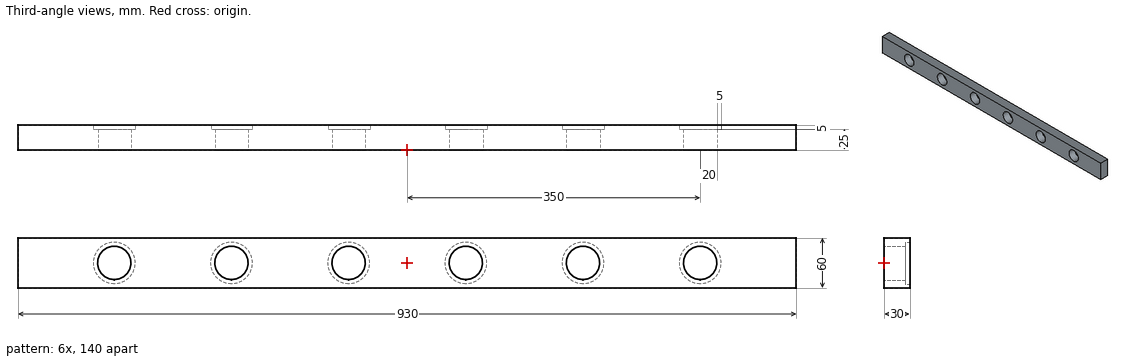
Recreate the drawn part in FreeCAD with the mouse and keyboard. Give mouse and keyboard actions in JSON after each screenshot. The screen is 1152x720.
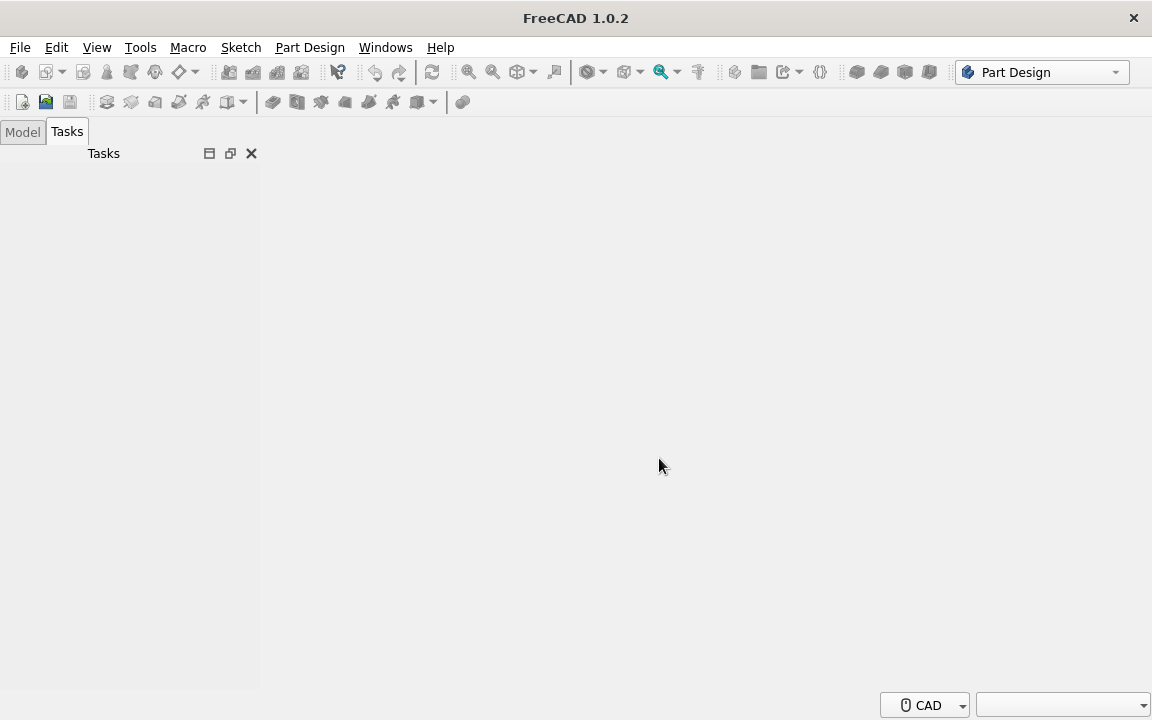
{"action": "left_click", "coordinate": [22, 102]}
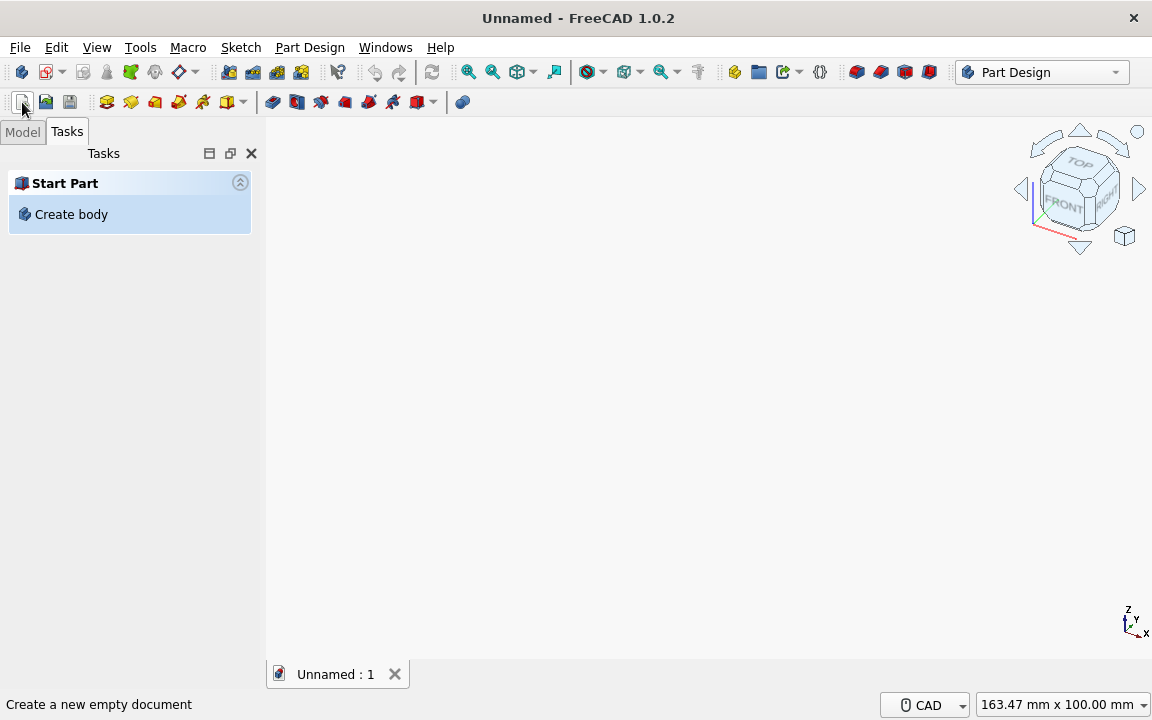
{"action": "left_click", "coordinate": [46, 72]}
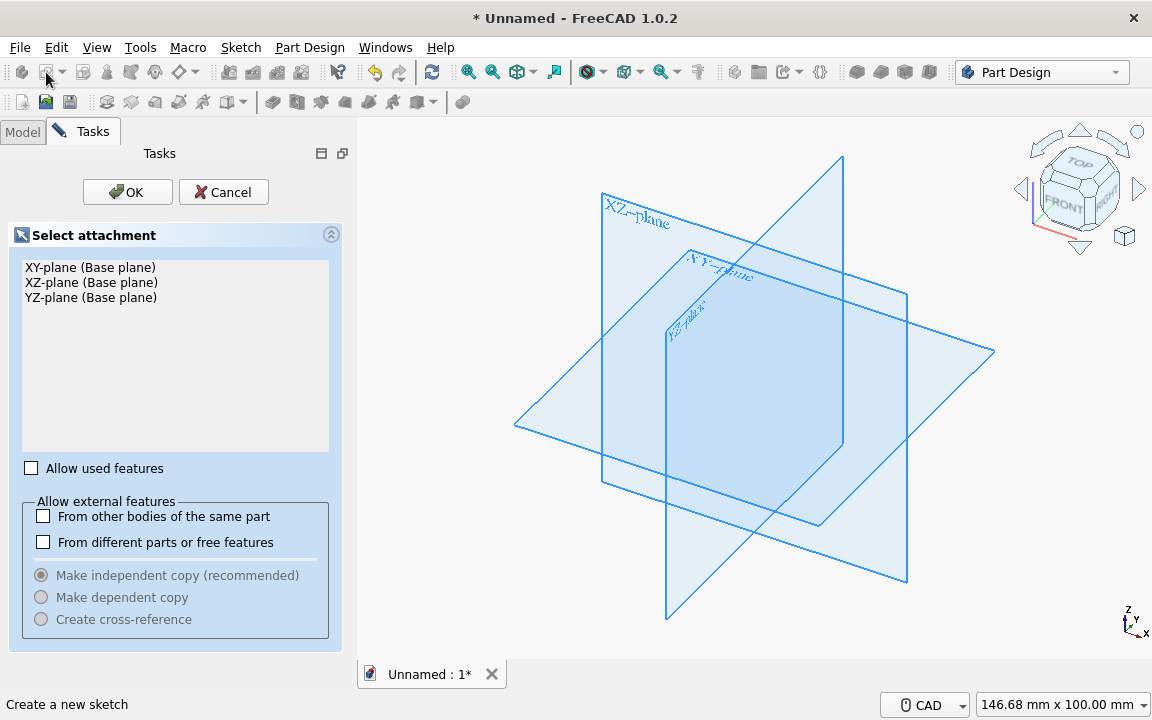
{"action": "left_click", "coordinate": [82, 282]}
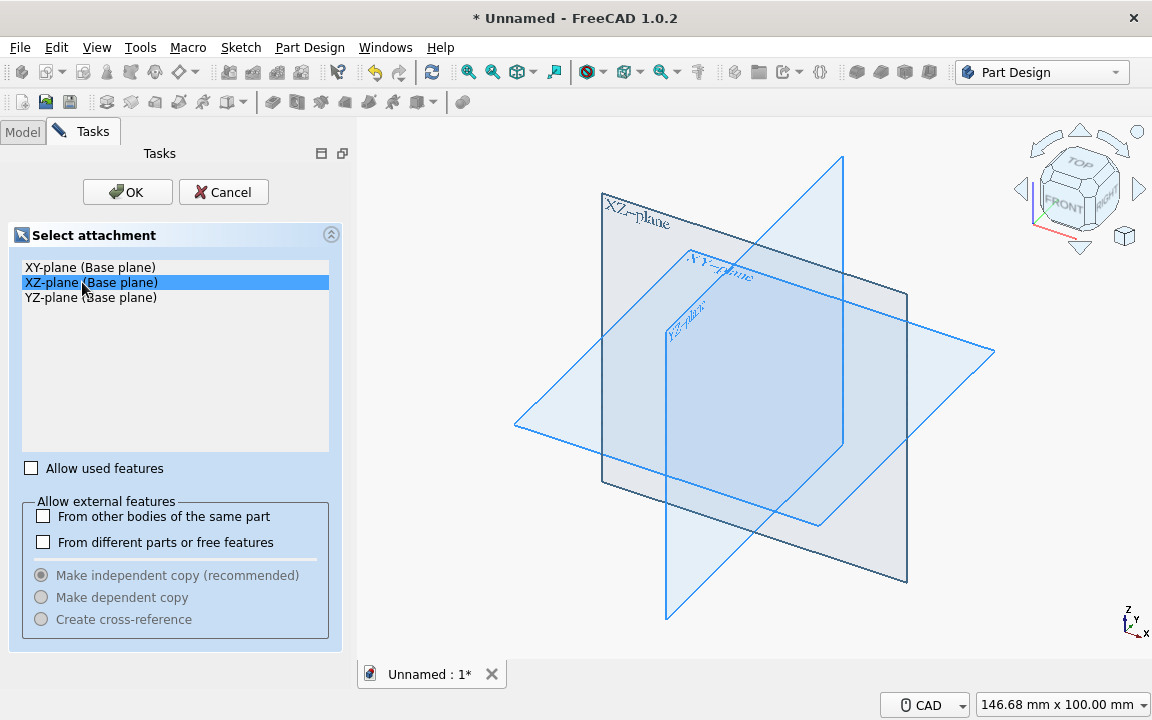
{"action": "left_click", "coordinate": [128, 192]}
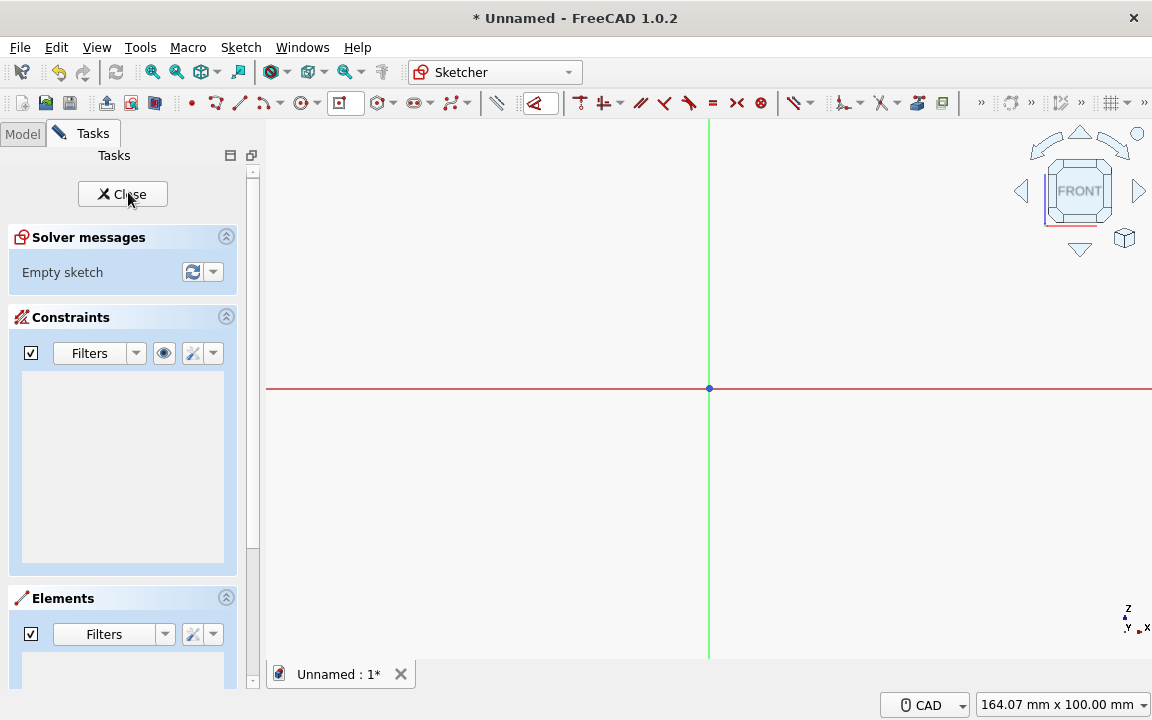
{"action": "scroll", "coordinate": [634, 389], "scroll_direction": "down", "scroll_amount": 12}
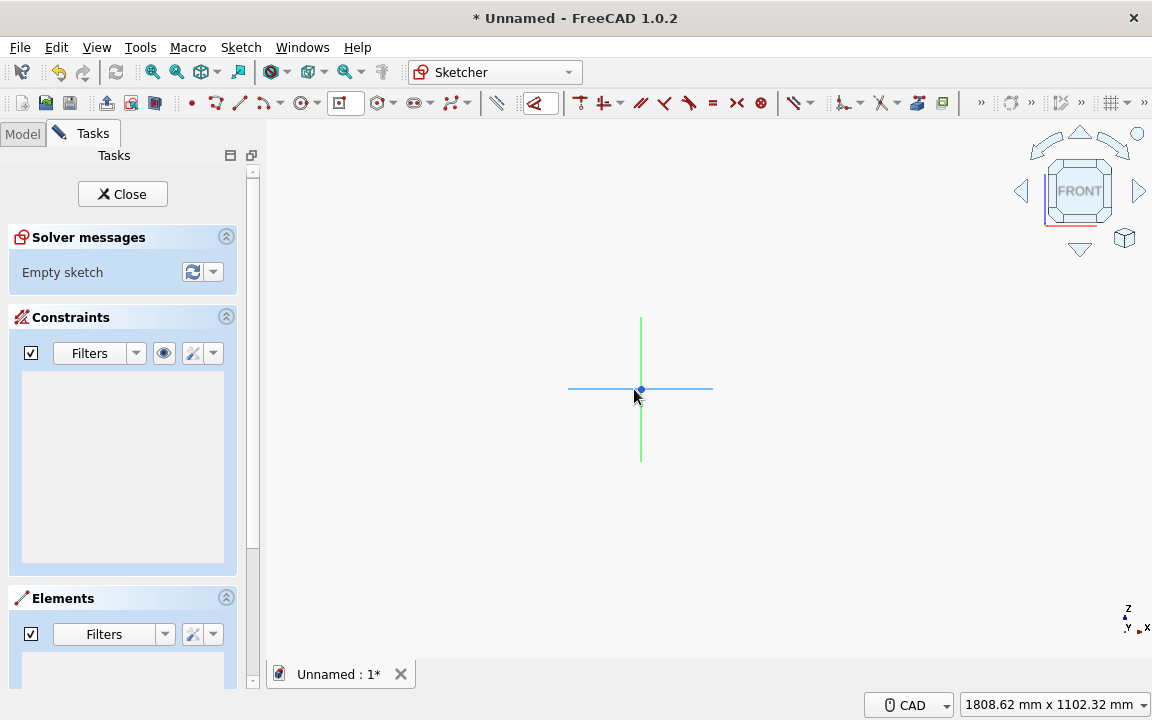
{"action": "left_click", "coordinate": [340, 104]}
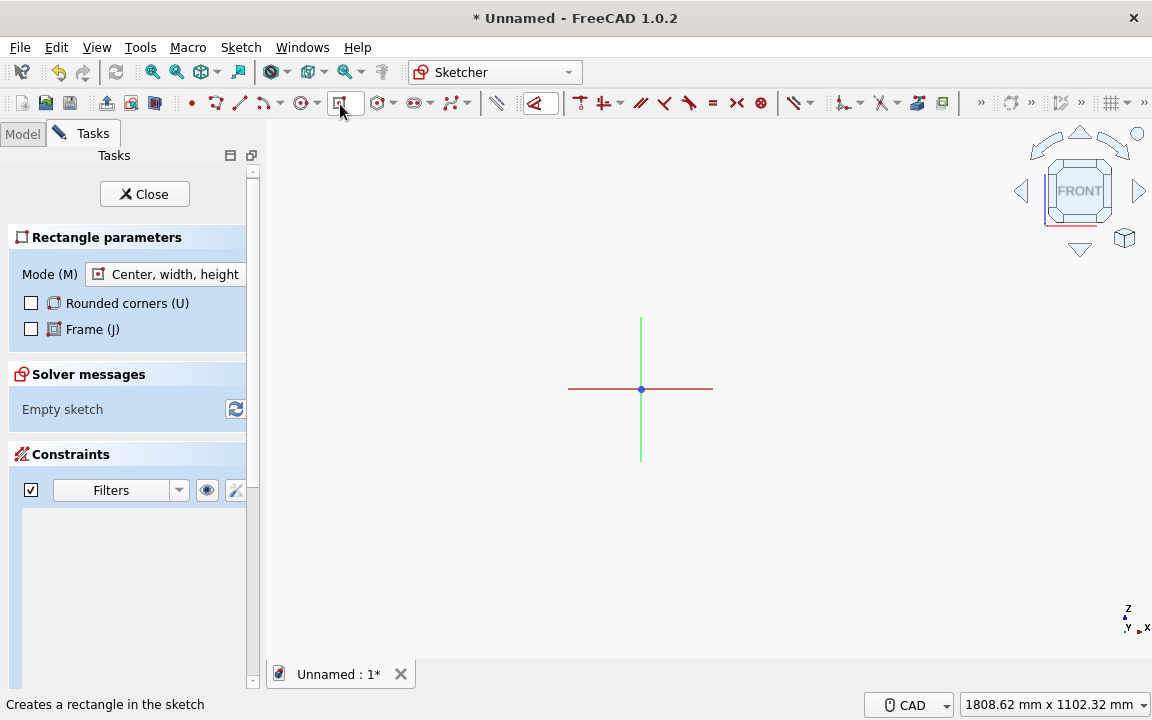
{"action": "left_click", "coordinate": [641, 389]}
{"action": "left_click", "coordinate": [869, 375]}
{"action": "key", "text": "Escape"}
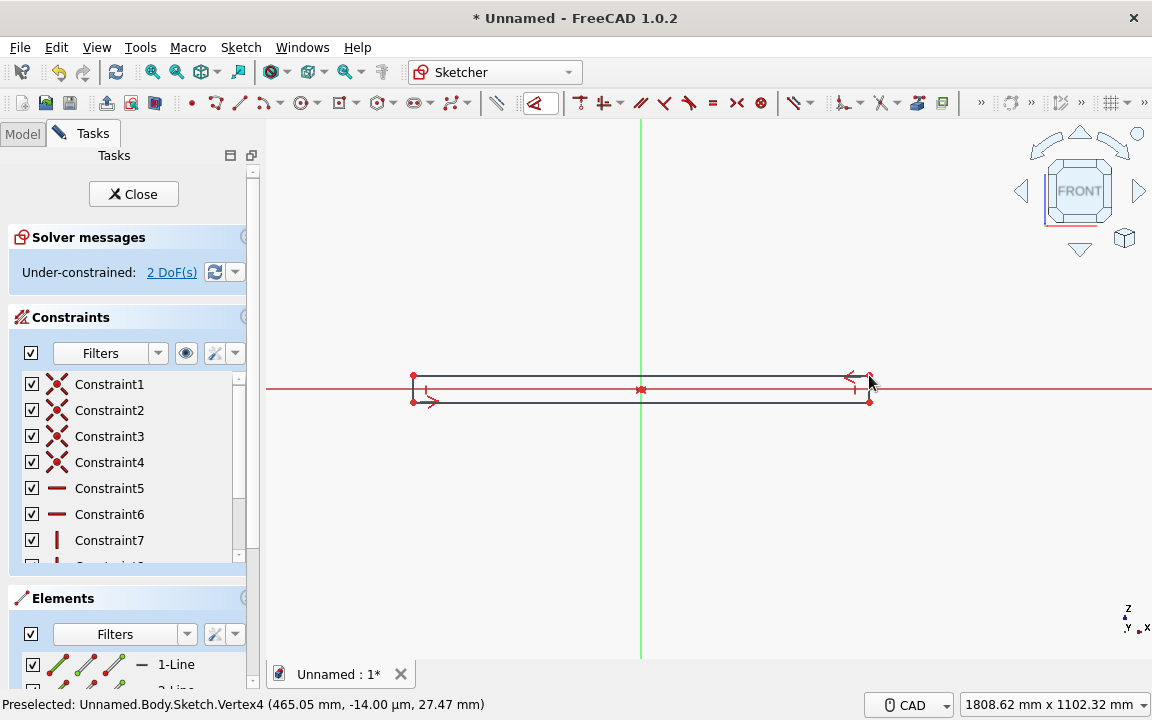
{"action": "left_click", "coordinate": [534, 104]}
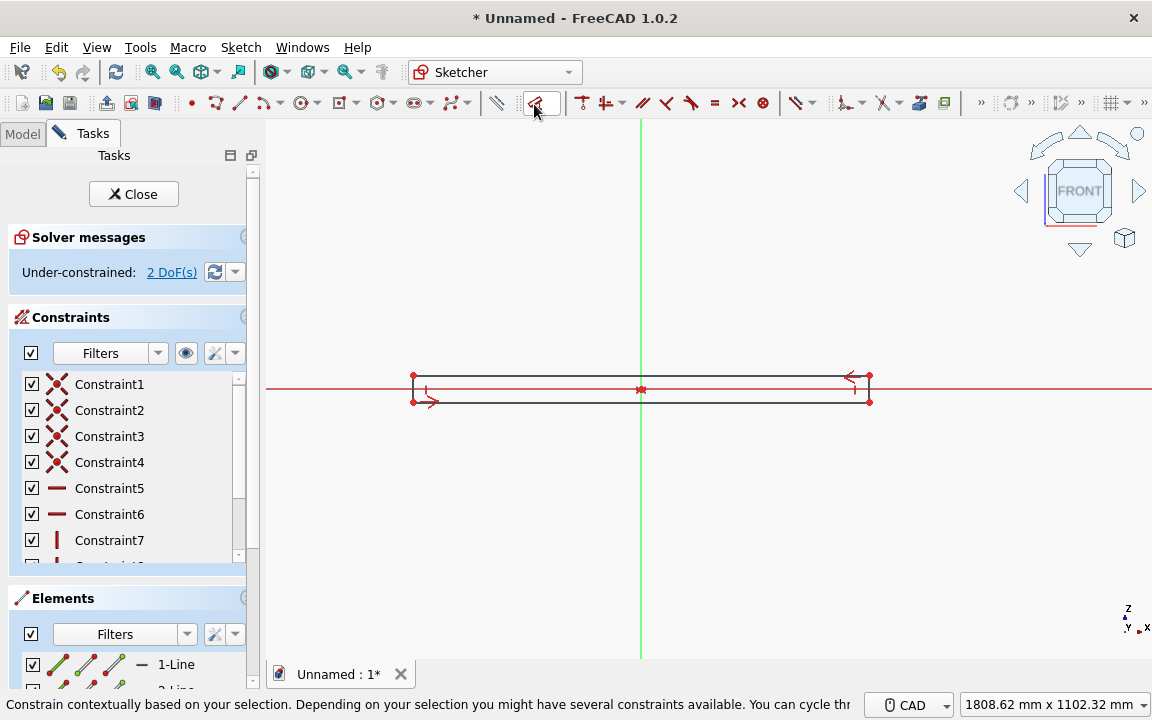
{"action": "scroll", "coordinate": [869, 392], "scroll_direction": "up", "scroll_amount": 2}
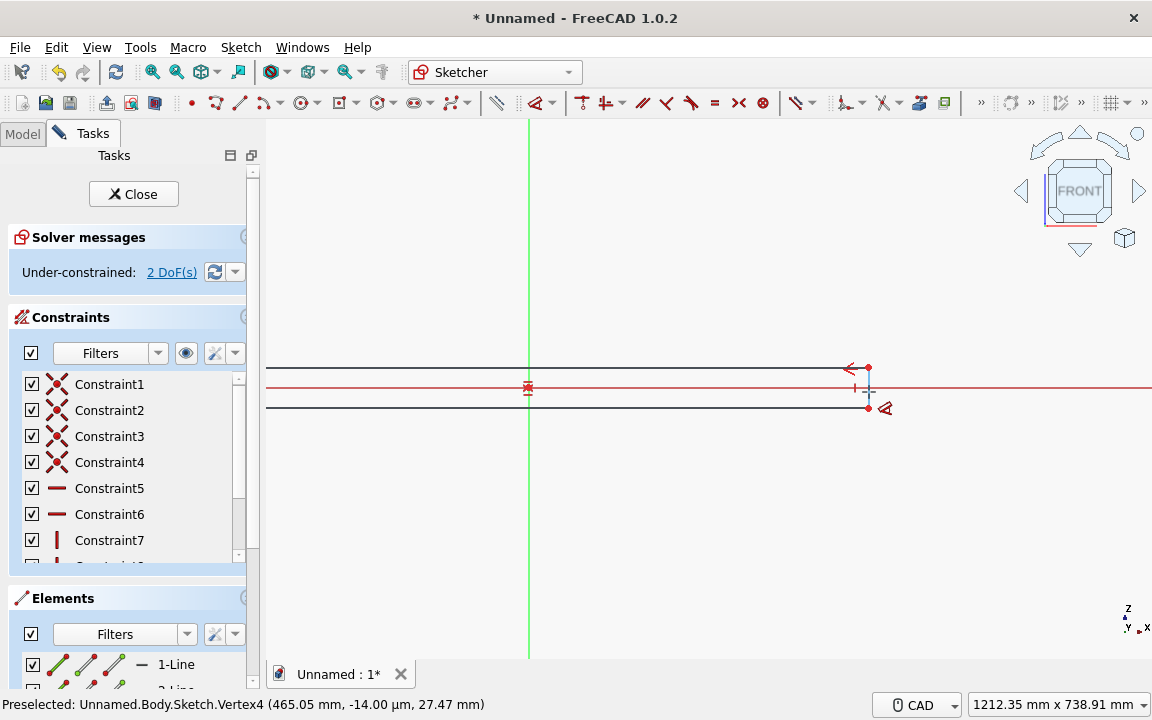
{"action": "left_click", "coordinate": [869, 392]}
{"action": "left_click", "coordinate": [903, 374]}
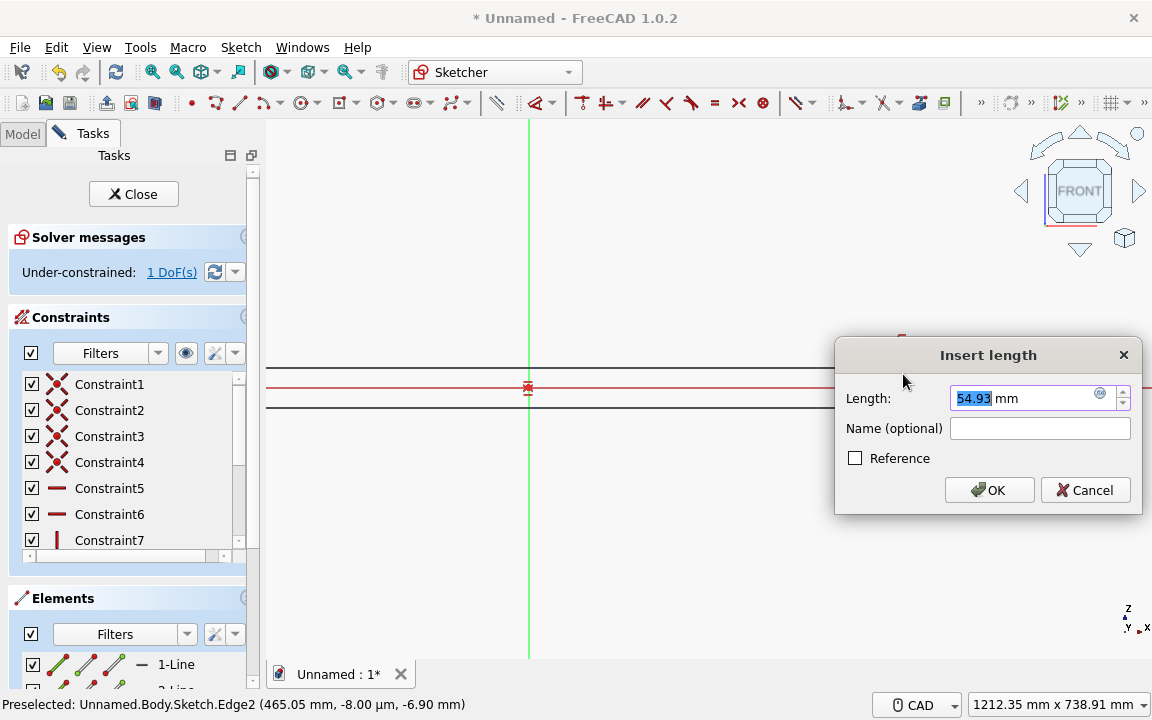
{"action": "type", "text": "60"}
{"action": "key", "text": "Return"}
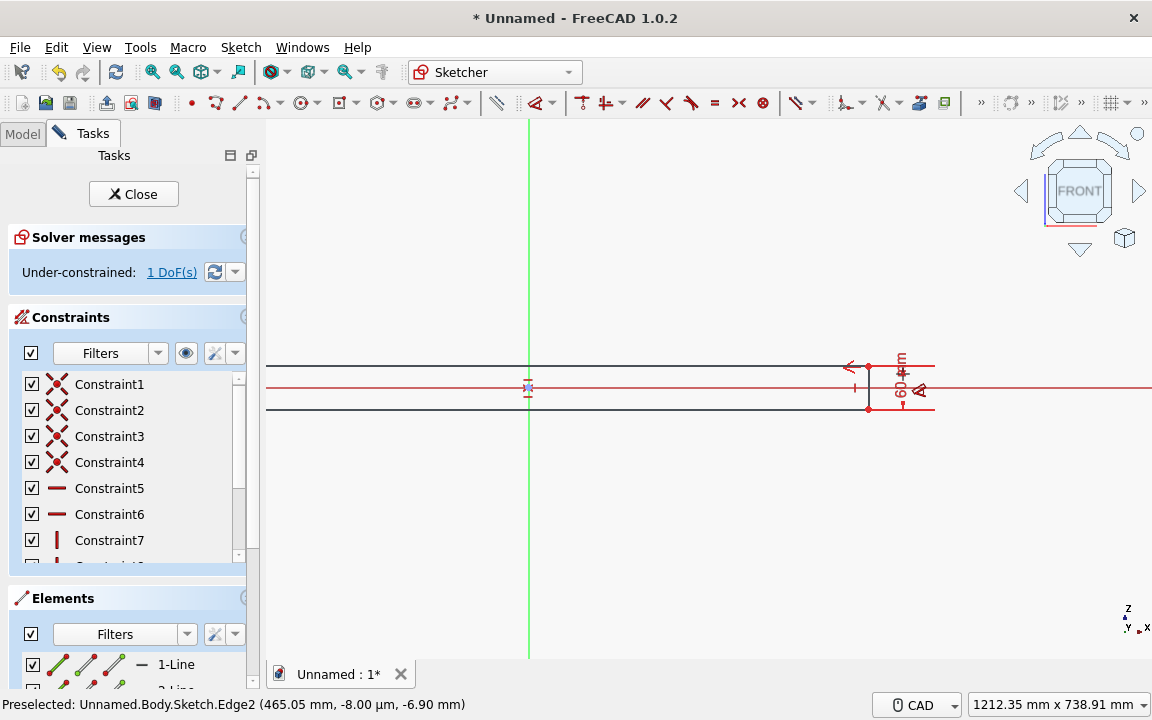
{"action": "left_click", "coordinate": [393, 410]}
{"action": "left_click", "coordinate": [581, 444]}